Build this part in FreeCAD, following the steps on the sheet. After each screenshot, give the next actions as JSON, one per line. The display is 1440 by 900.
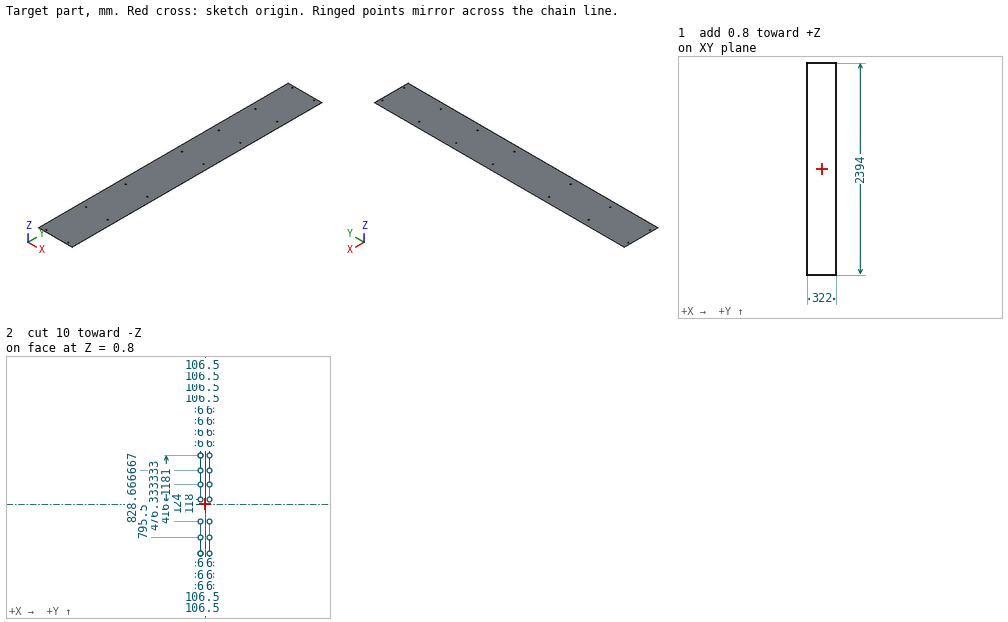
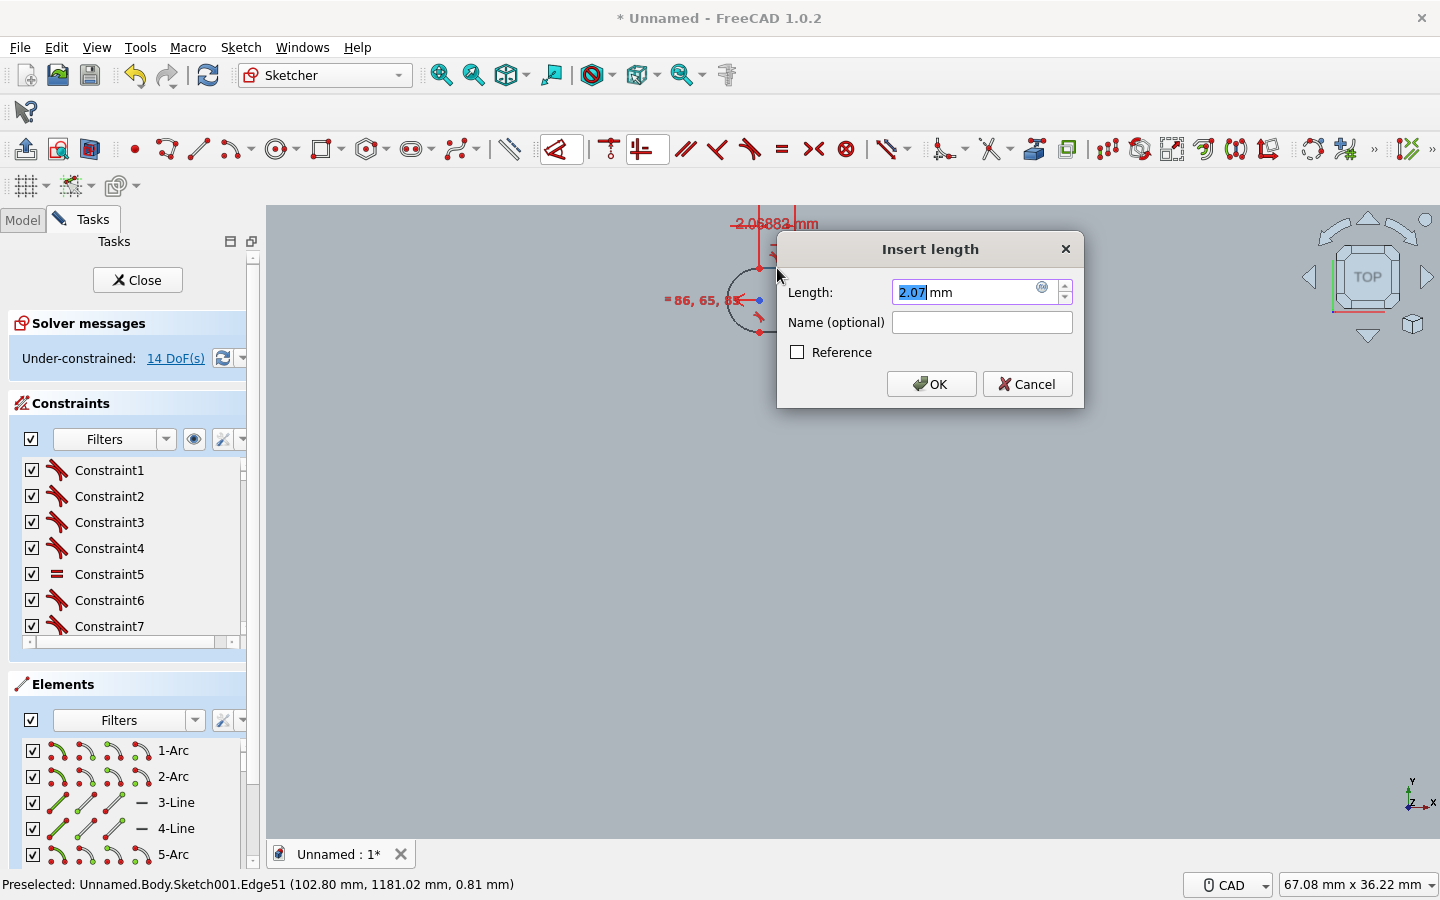
{"action": "type", "text": "6"}
{"action": "key", "text": "Return"}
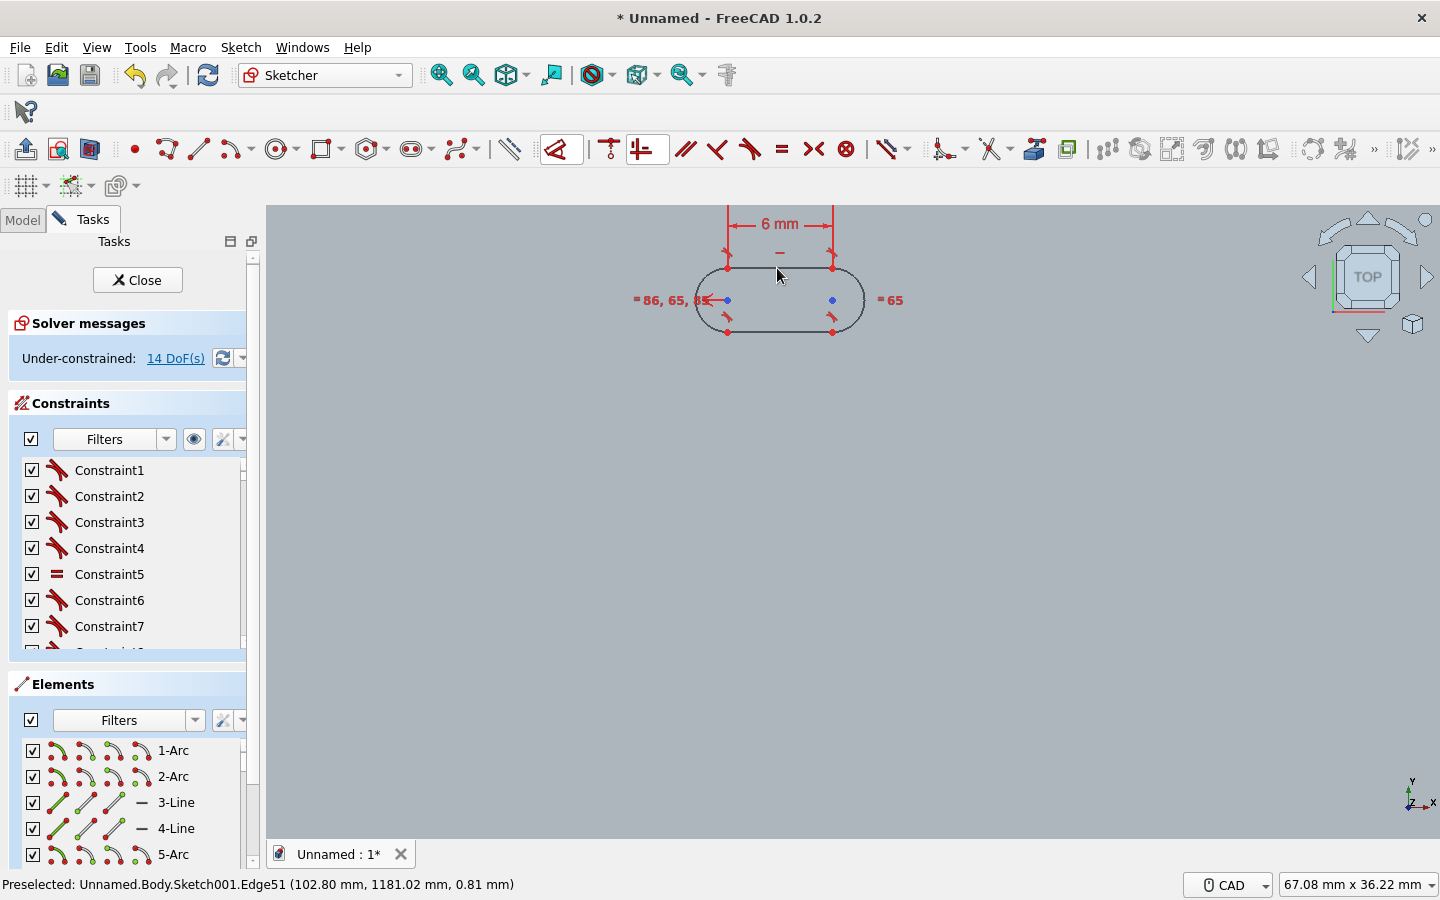
{"action": "scroll", "coordinate": [784, 522], "scroll_direction": "down", "scroll_amount": 15}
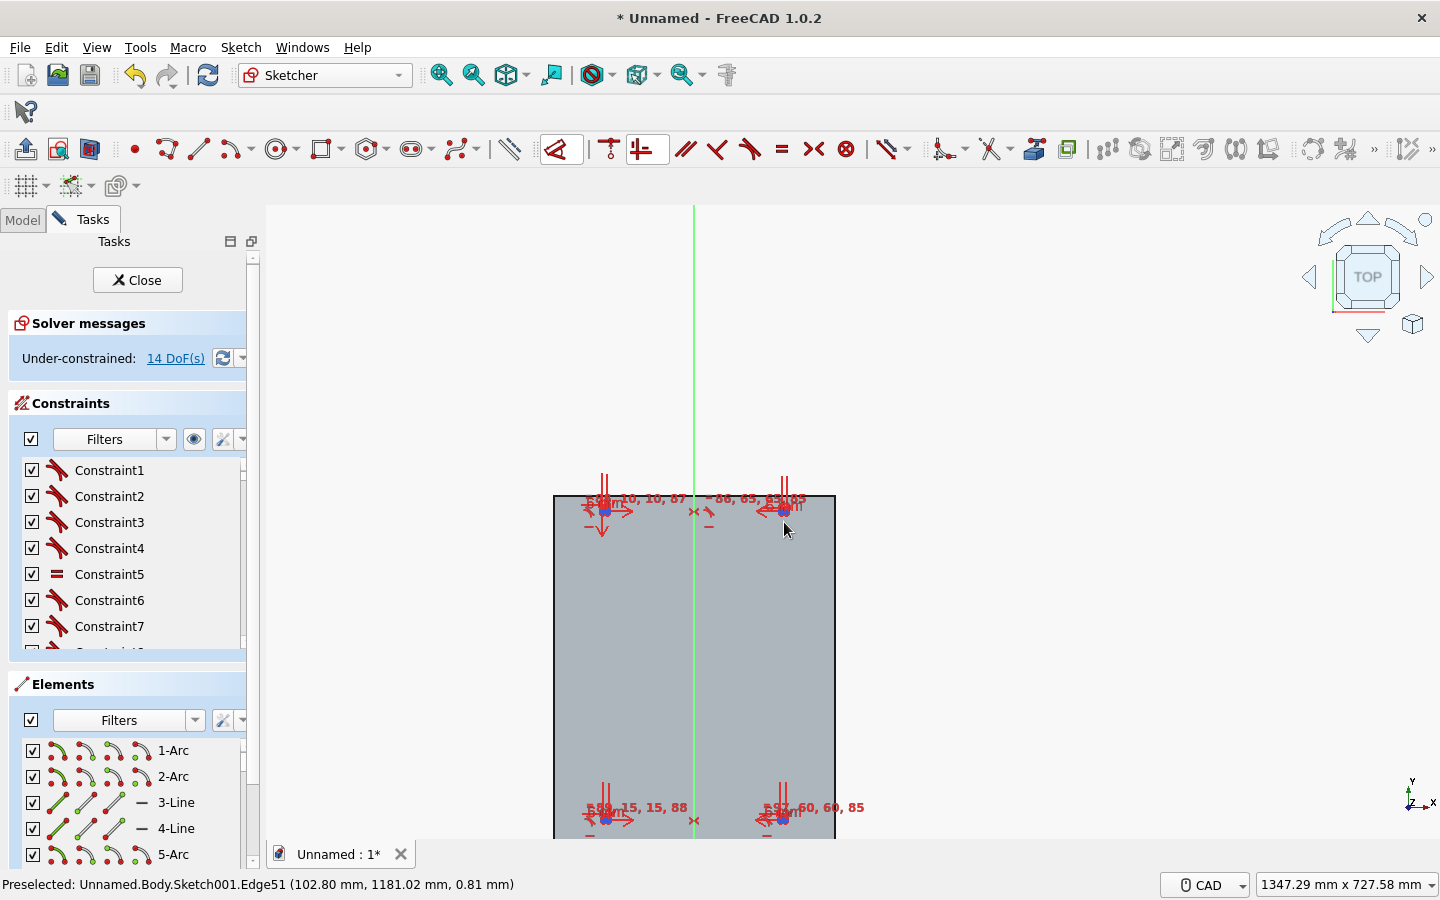
{"action": "scroll", "coordinate": [807, 265], "scroll_direction": "down", "scroll_amount": 8}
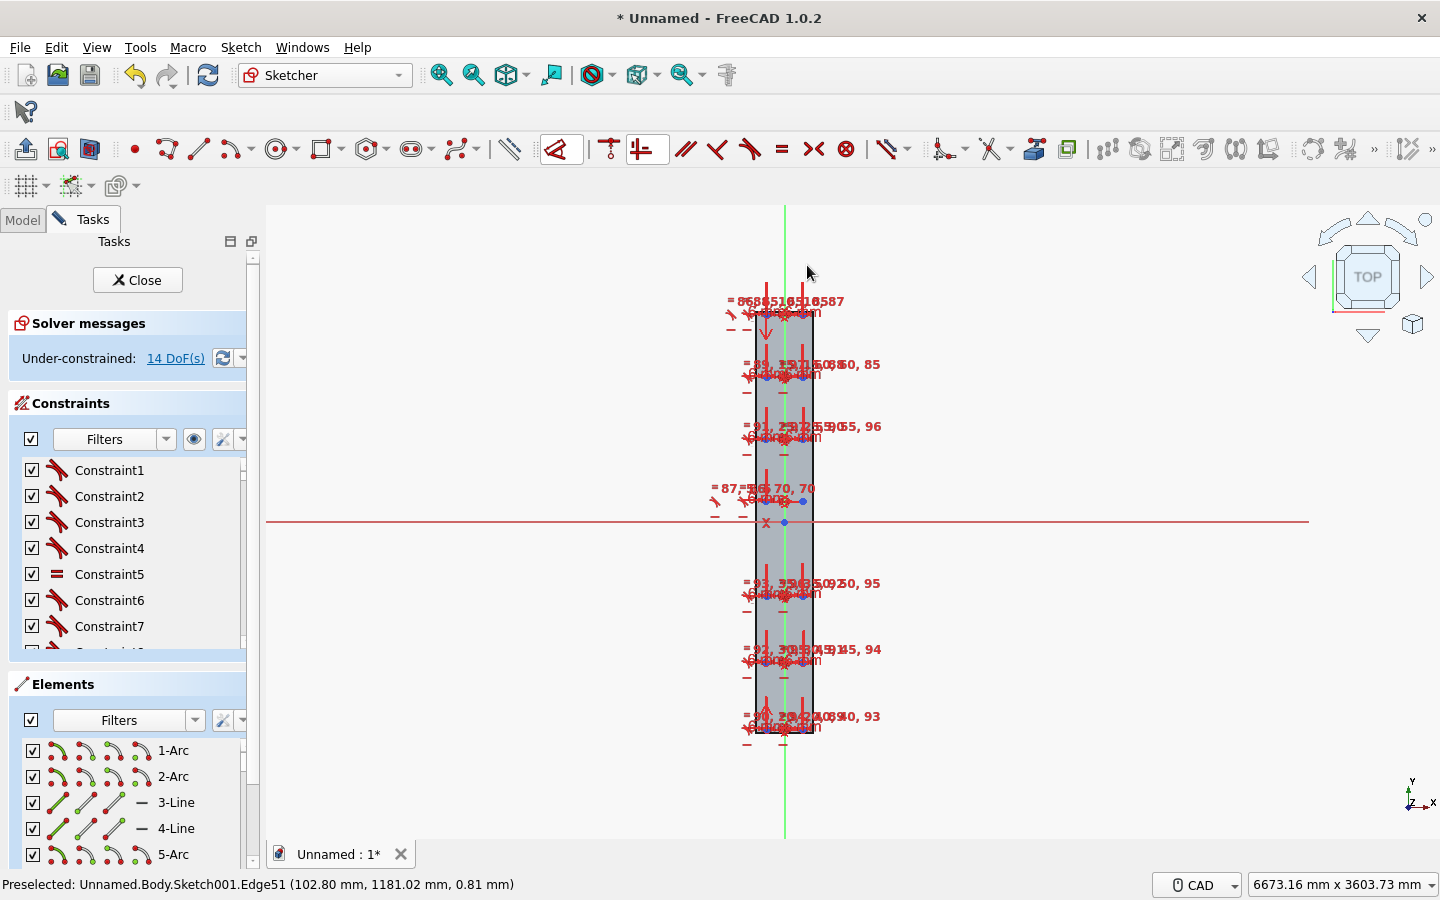
{"action": "scroll", "coordinate": [803, 501], "scroll_direction": "up", "scroll_amount": 19}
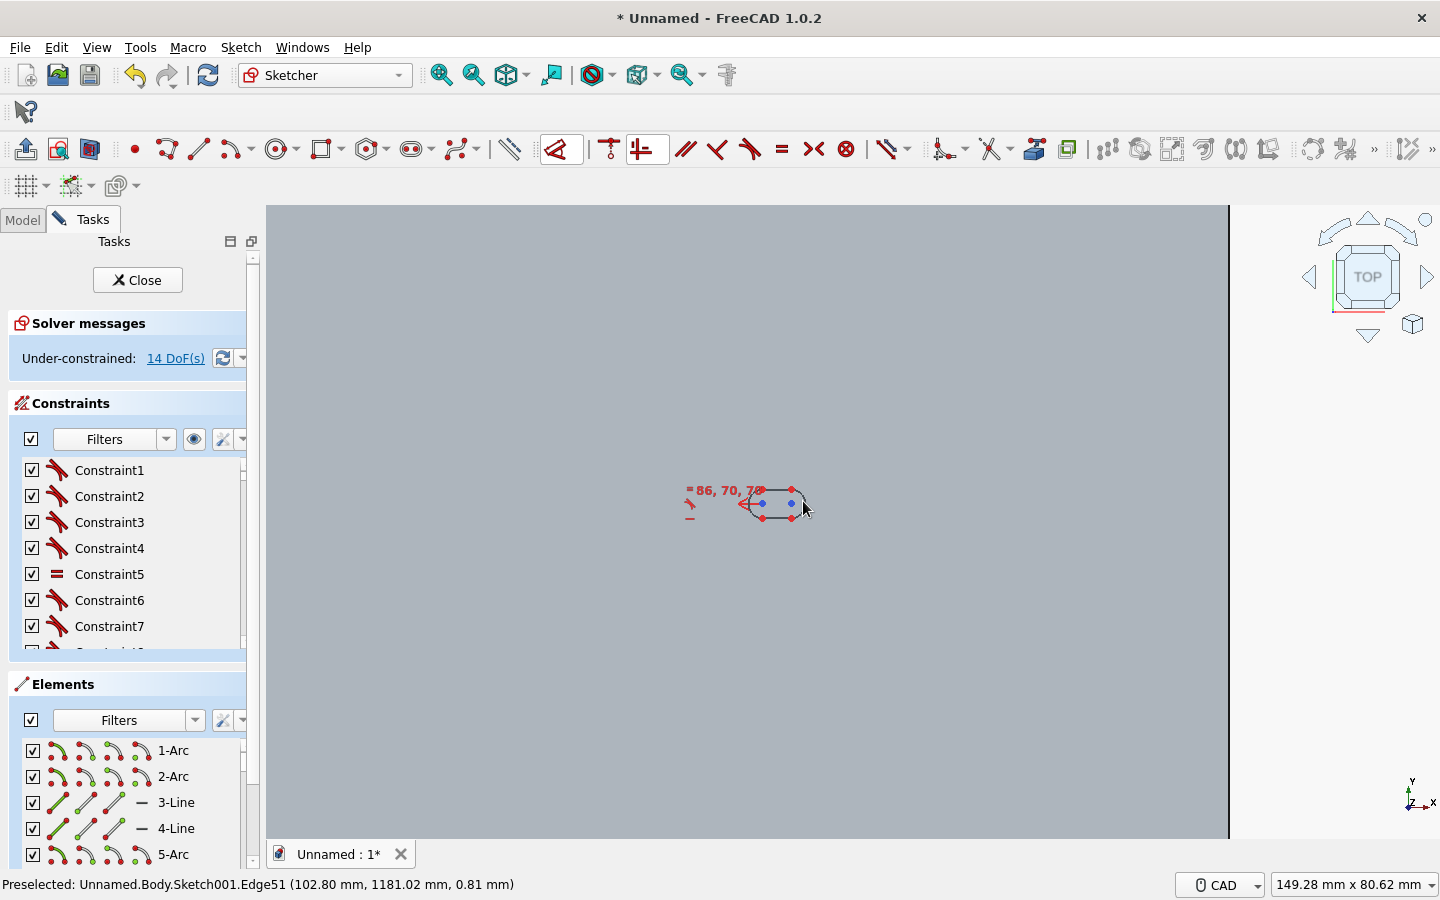
{"action": "left_click", "coordinate": [771, 490]}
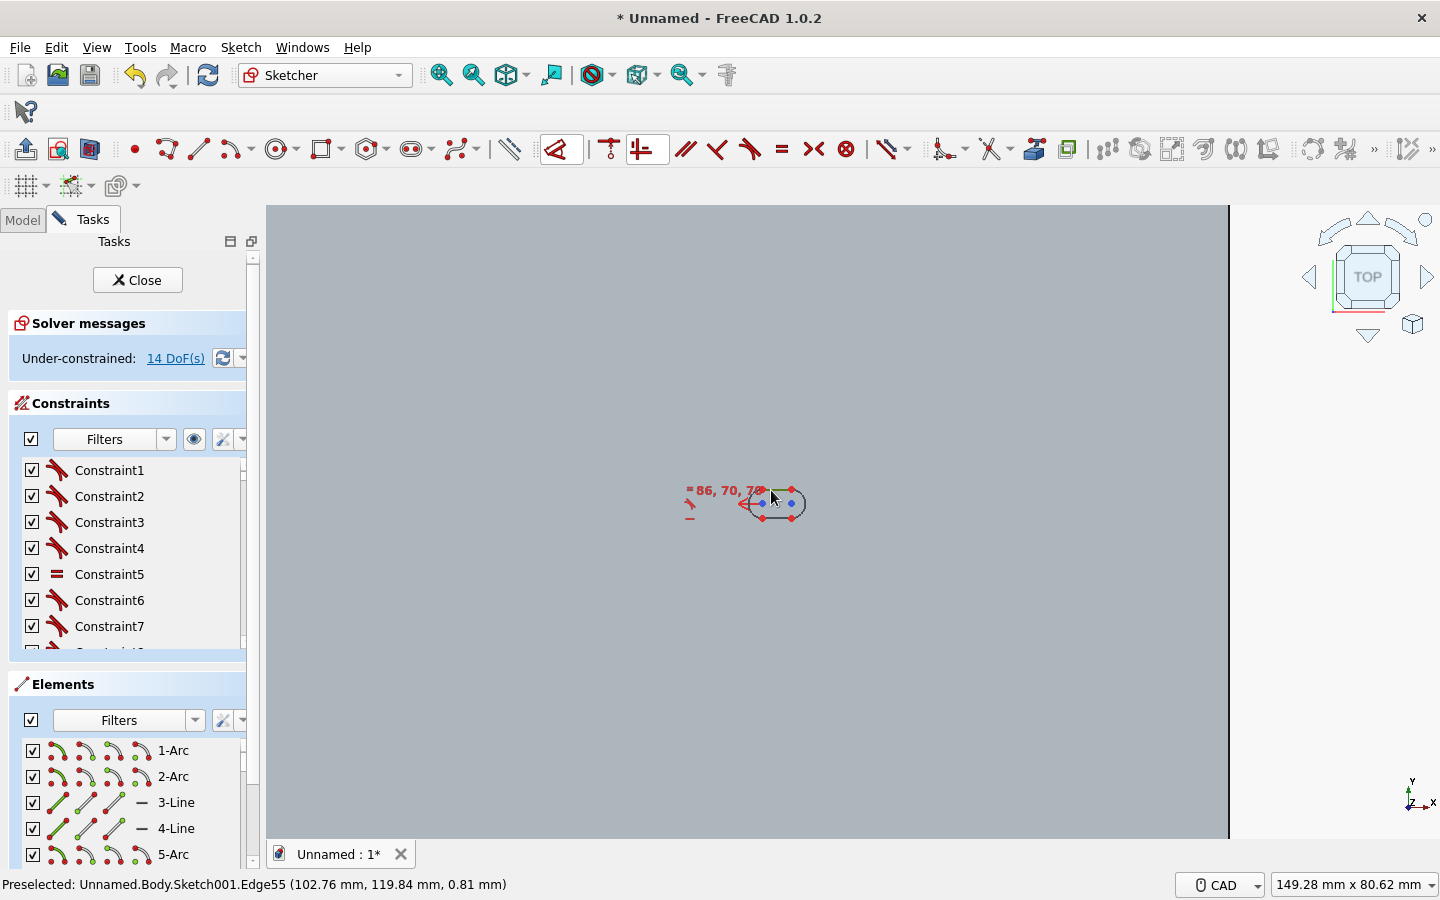
{"action": "key", "text": "l"}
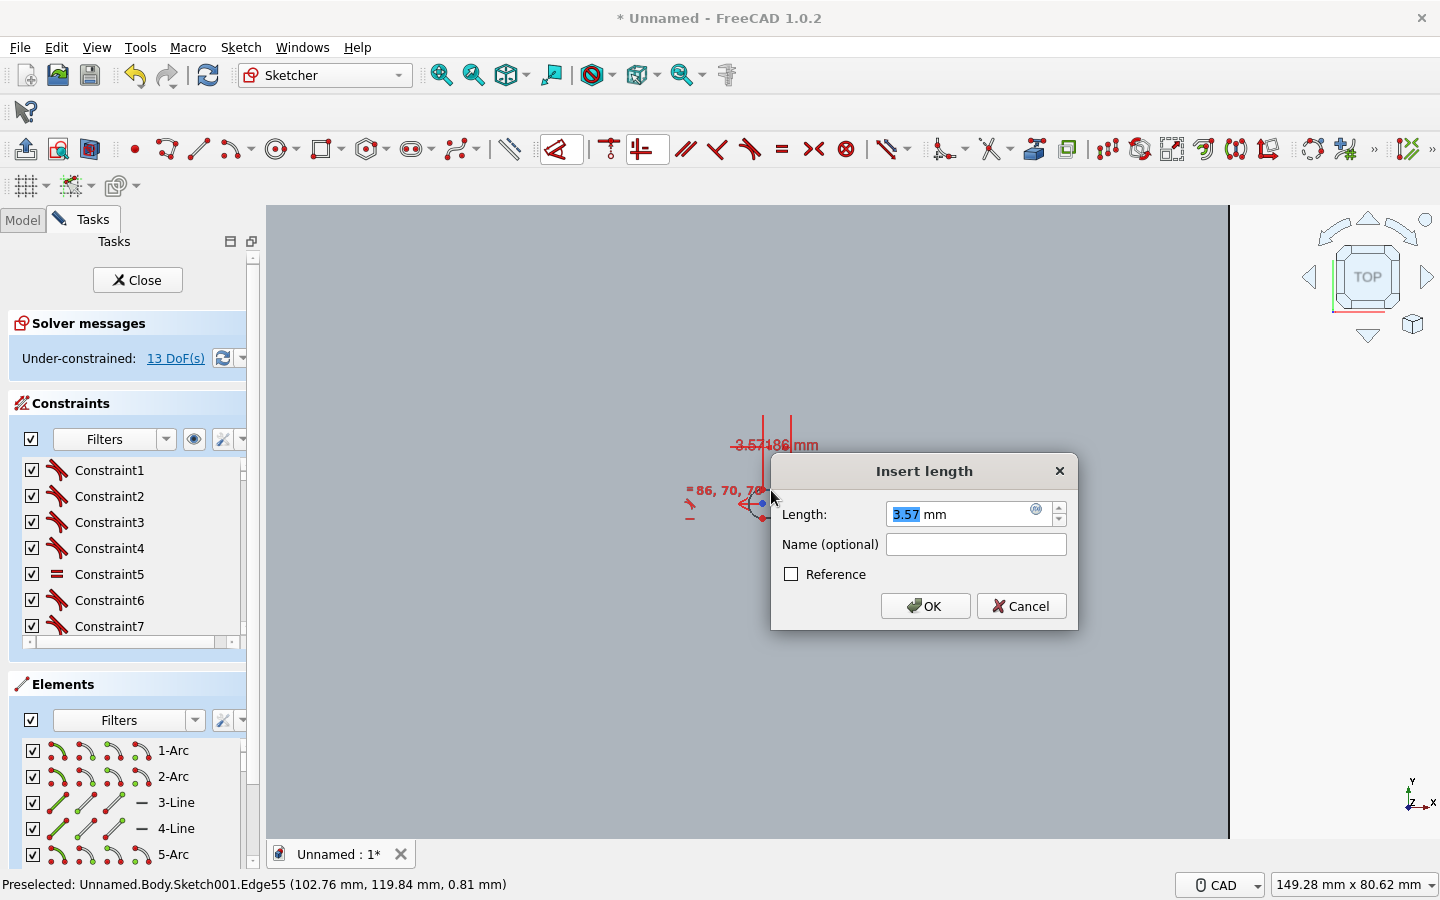
{"action": "type", "text": "6"}
{"action": "key", "text": "Return"}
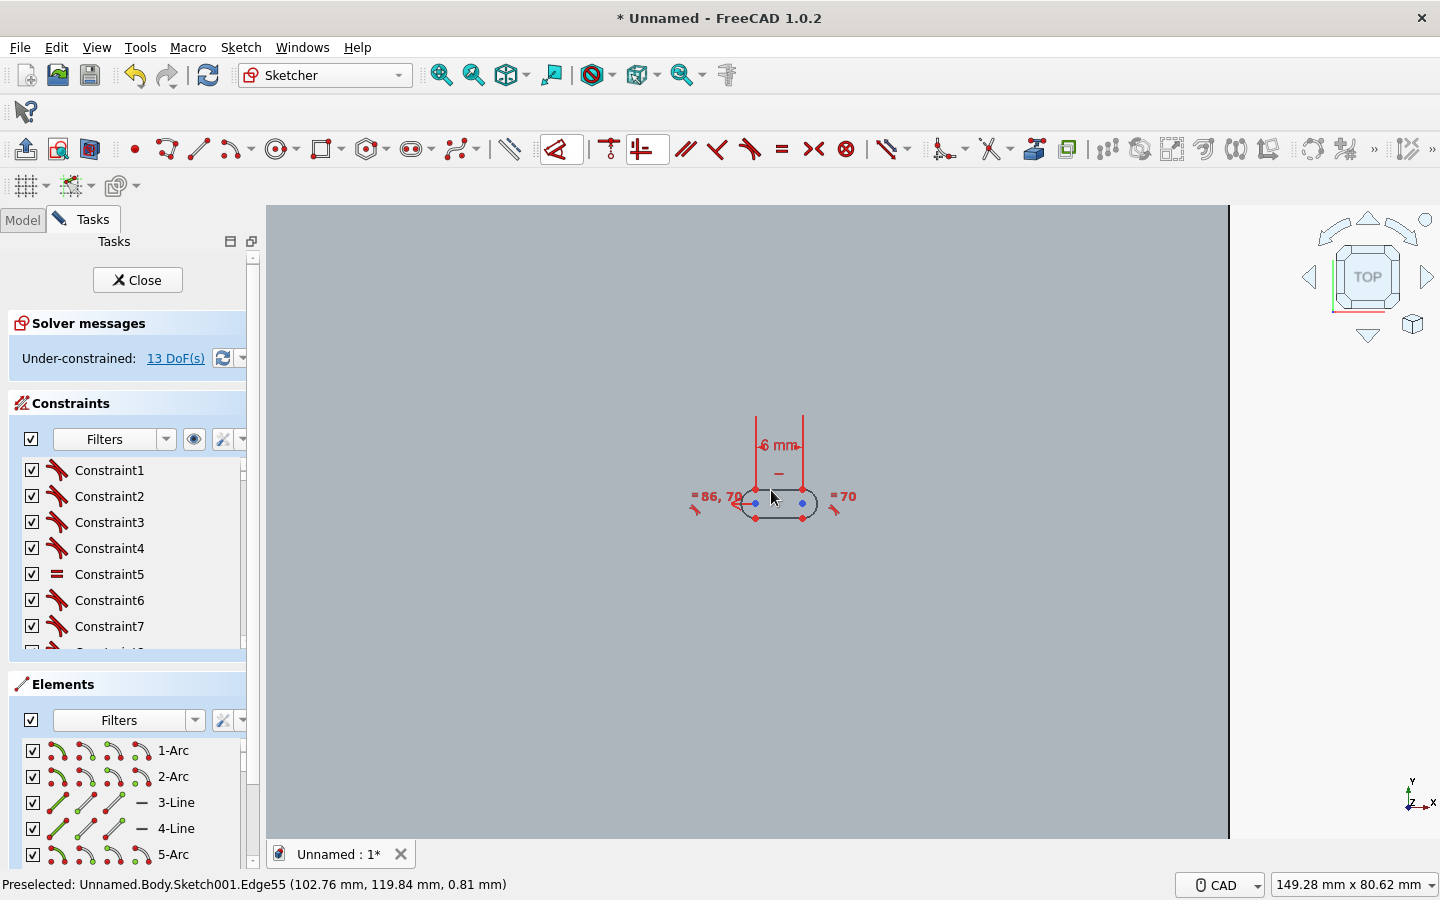
{"action": "scroll", "coordinate": [808, 496], "scroll_direction": "down", "scroll_amount": 18}